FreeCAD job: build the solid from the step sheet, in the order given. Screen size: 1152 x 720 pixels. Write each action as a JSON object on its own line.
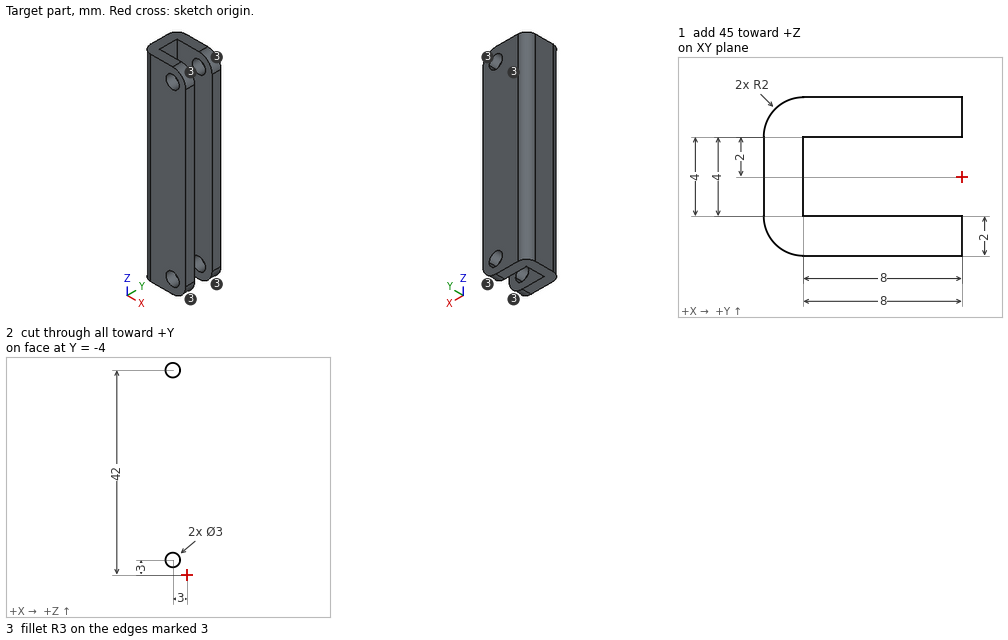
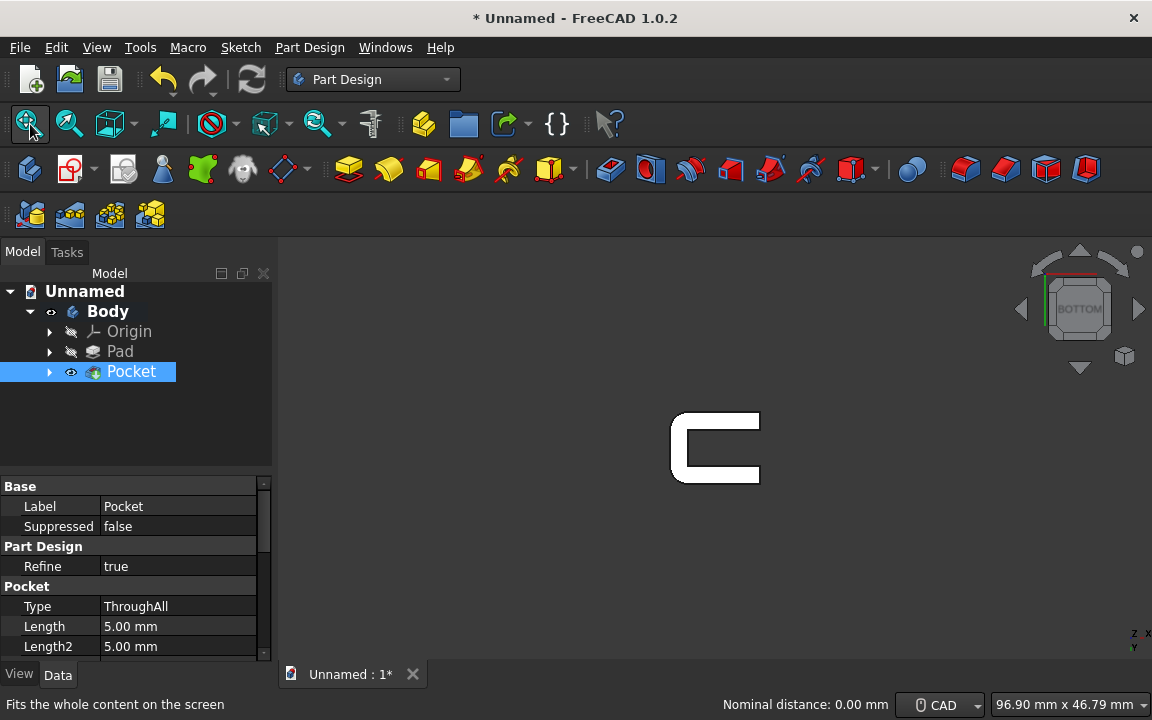
{"action": "left_click", "coordinate": [30, 124]}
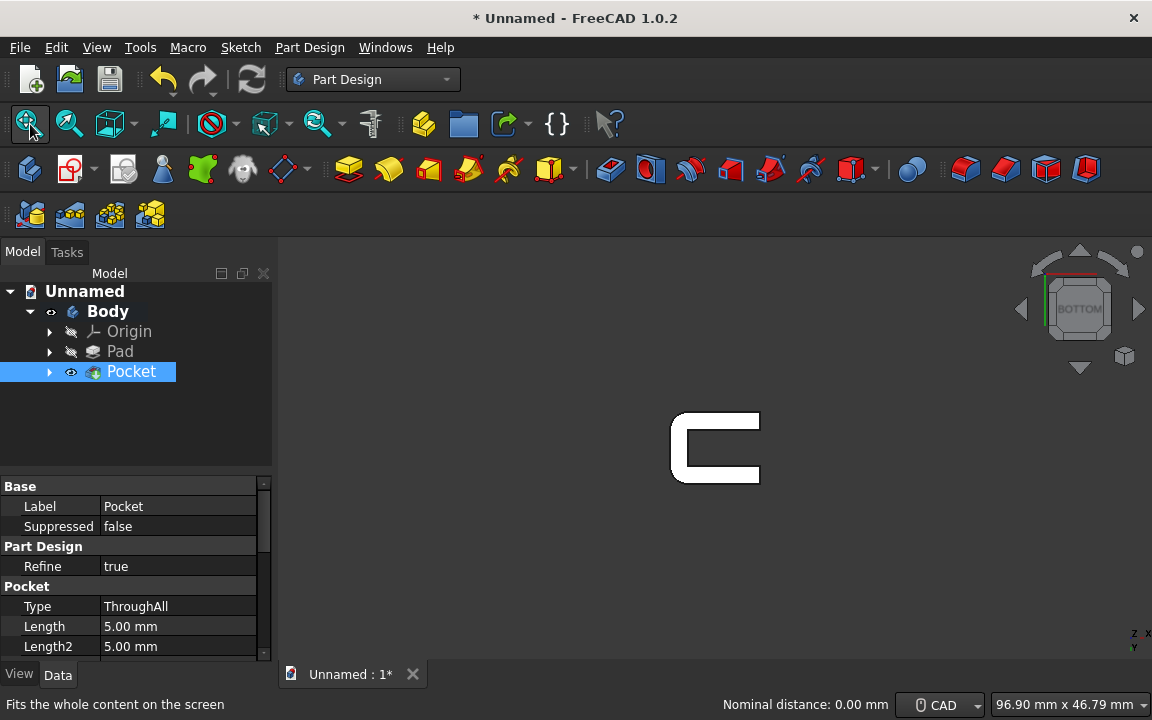
{"action": "left_click", "coordinate": [760, 474], "text": "ctrl"}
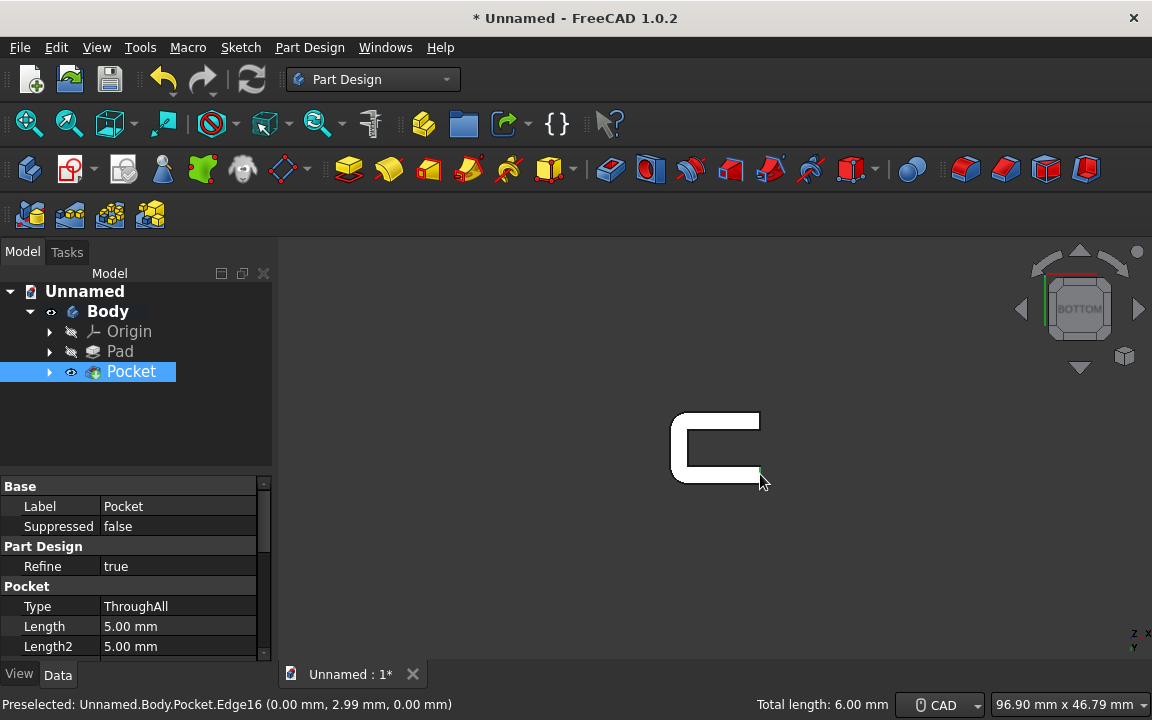
{"action": "left_click", "coordinate": [760, 420], "text": "ctrl"}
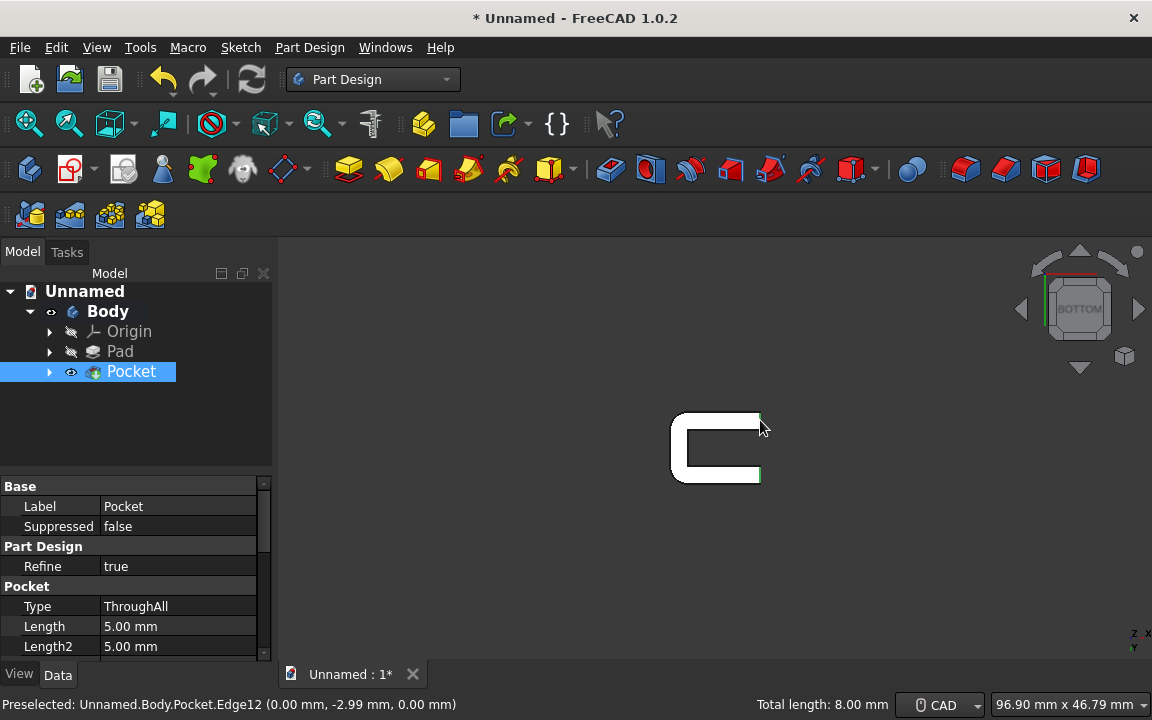
{"action": "left_click", "coordinate": [966, 170]}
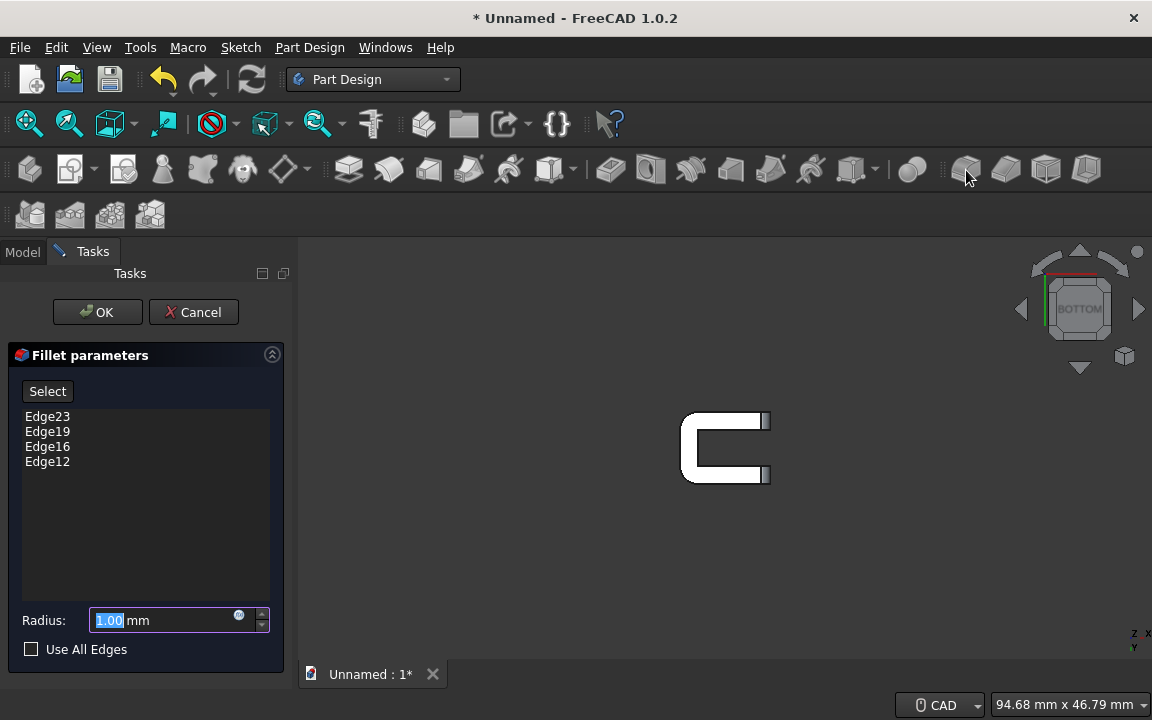
{"action": "type", "text": "3"}
{"action": "key", "text": "Tab"}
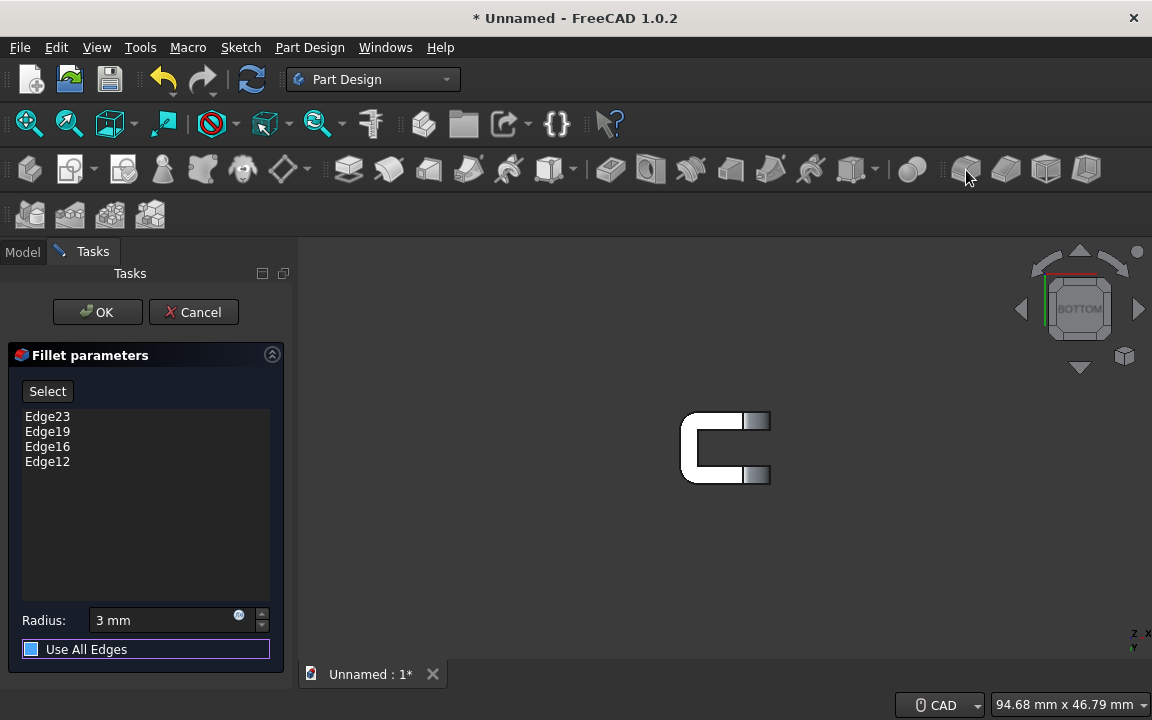
{"action": "left_click", "coordinate": [98, 312]}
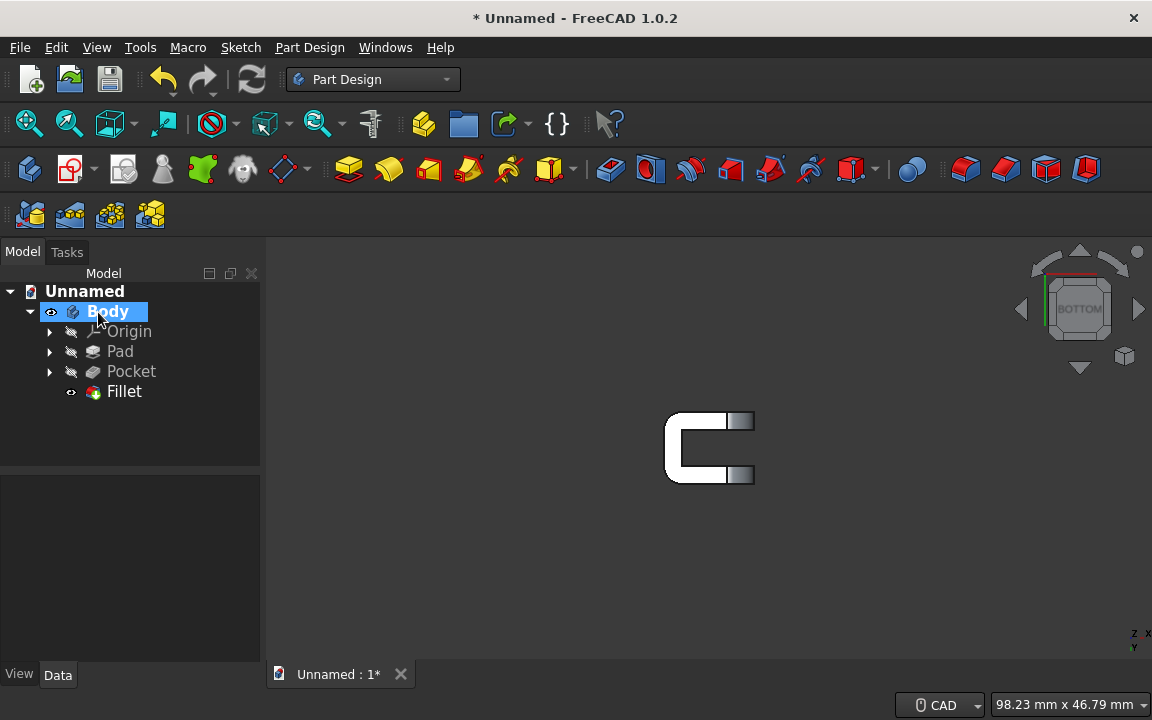
{"action": "key", "text": "0"}